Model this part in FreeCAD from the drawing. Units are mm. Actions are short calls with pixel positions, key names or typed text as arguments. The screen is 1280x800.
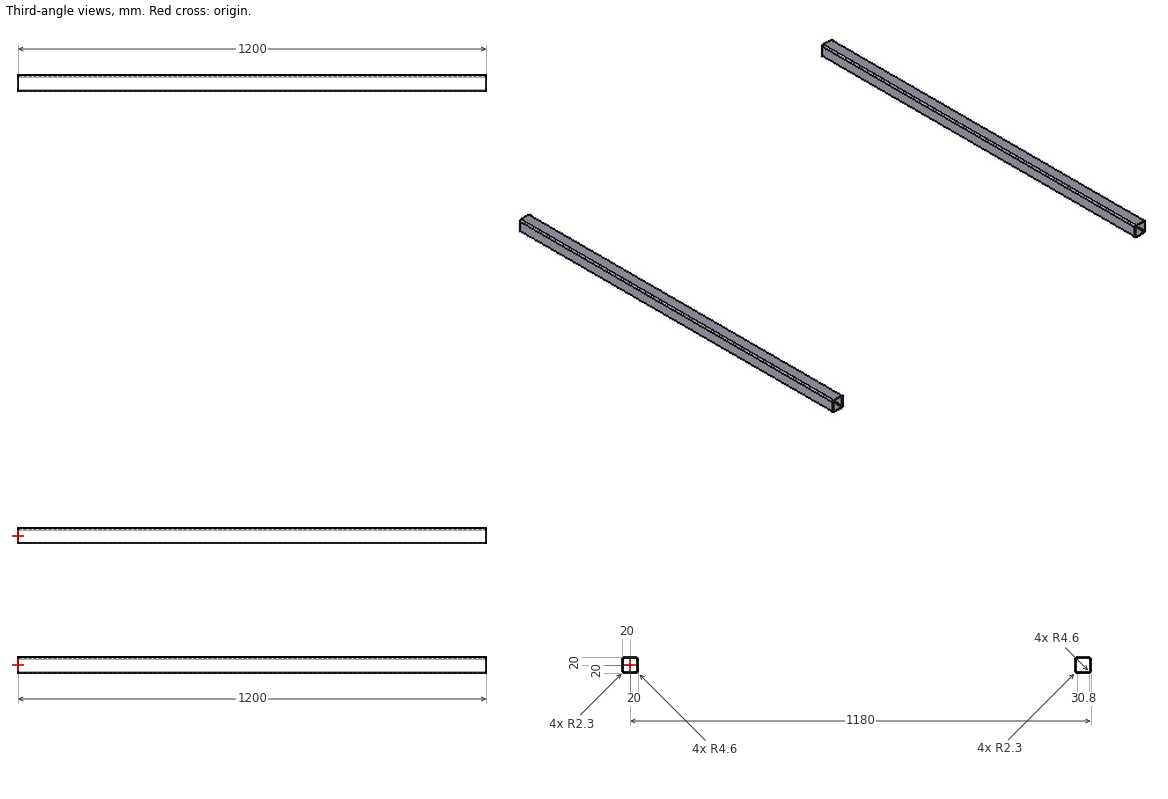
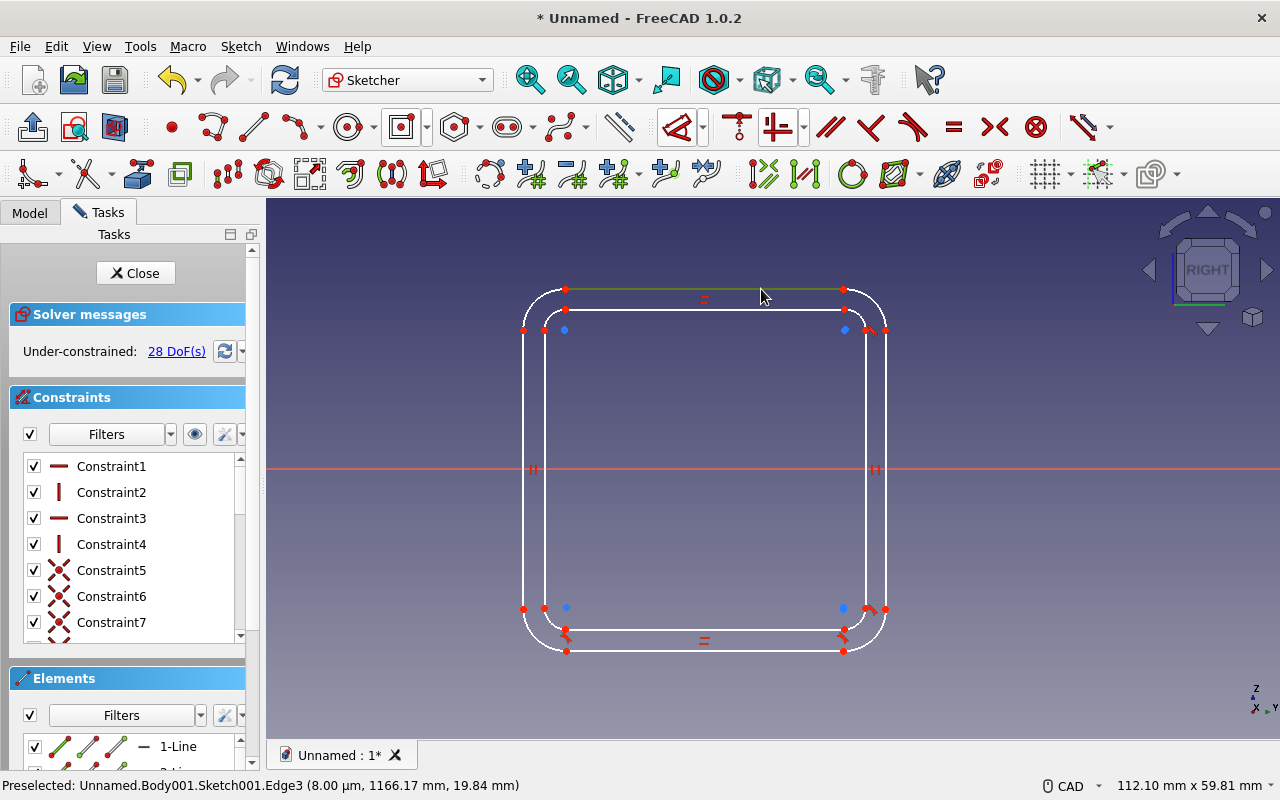
click(881, 311)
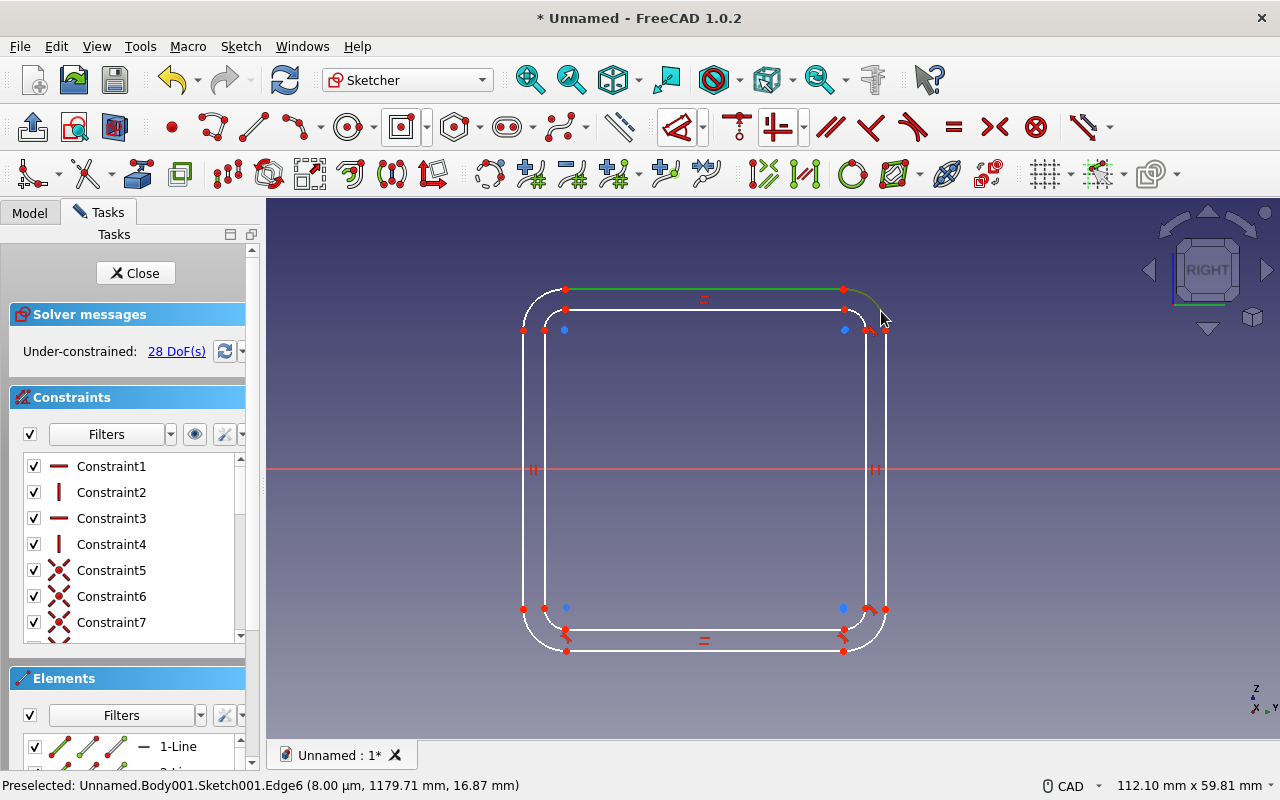
key(t)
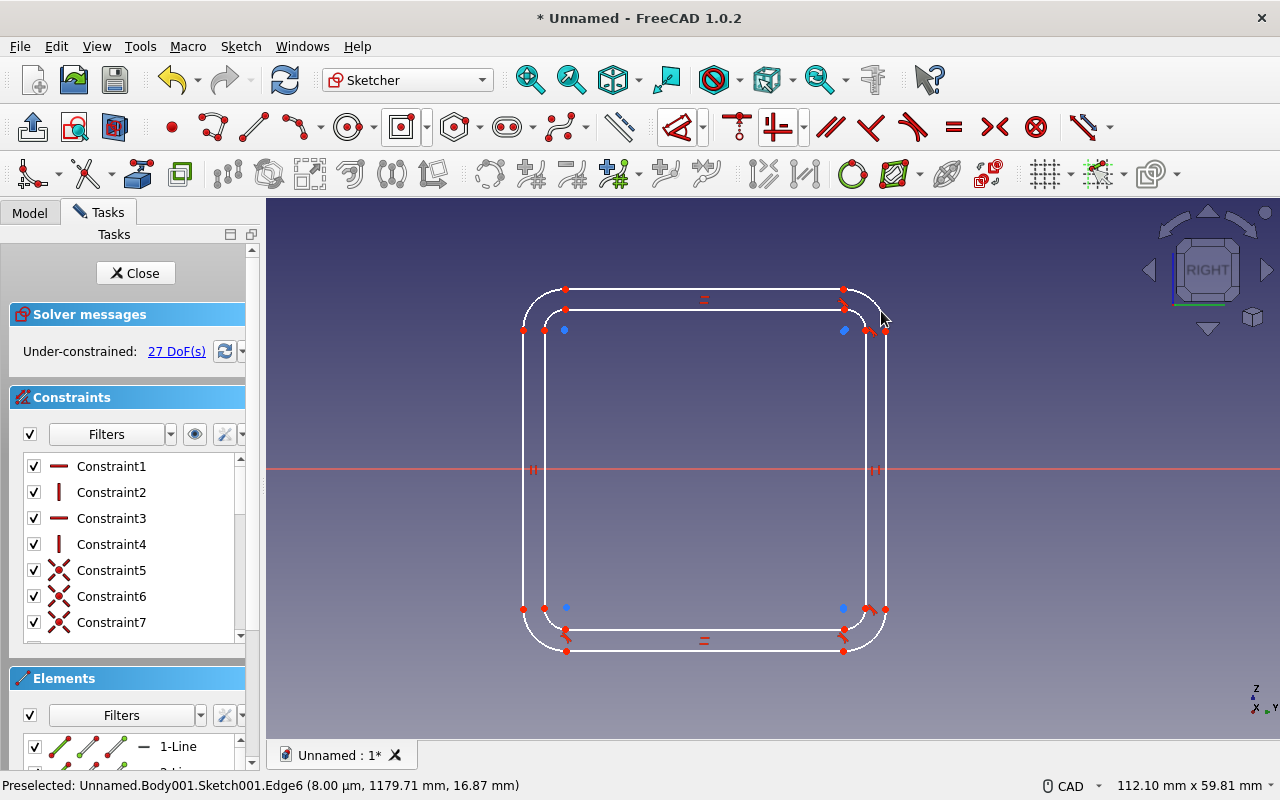
click(761, 289)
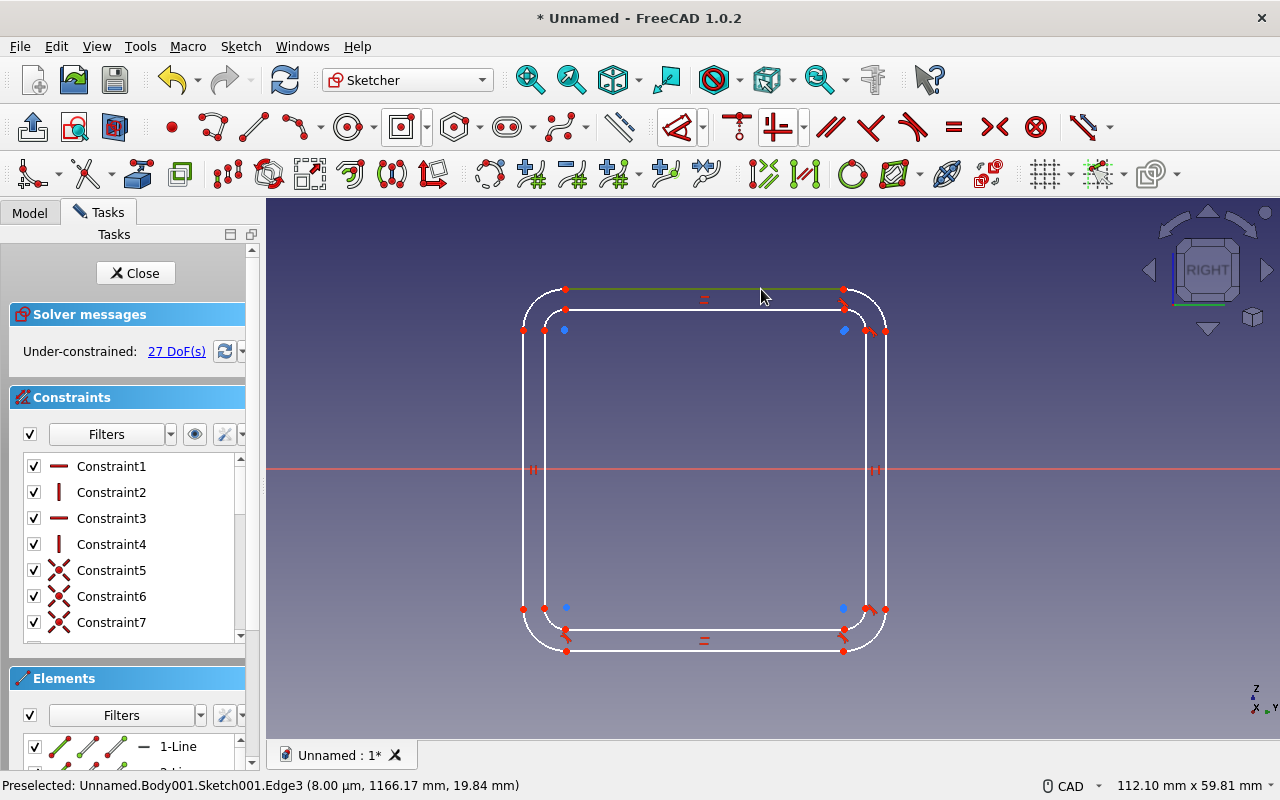
click(547, 293)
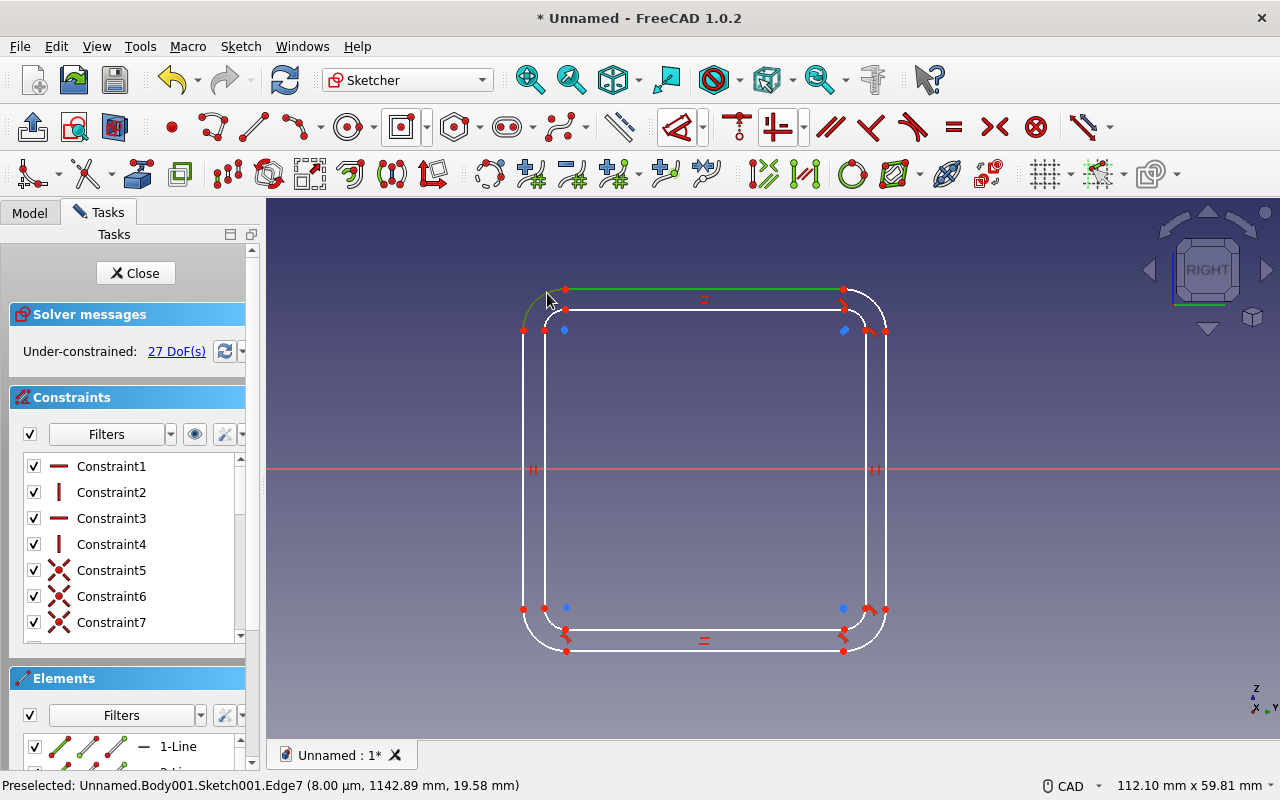
key(t)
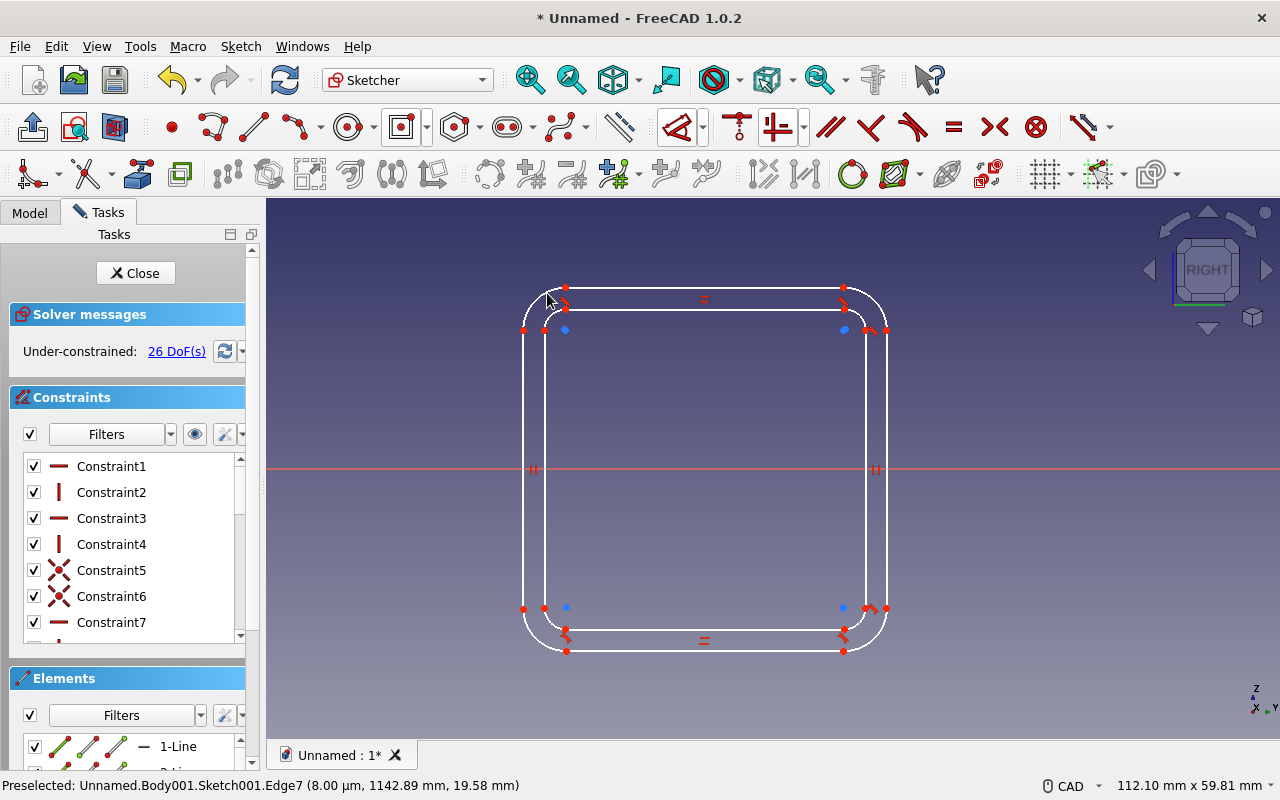
click(523, 414)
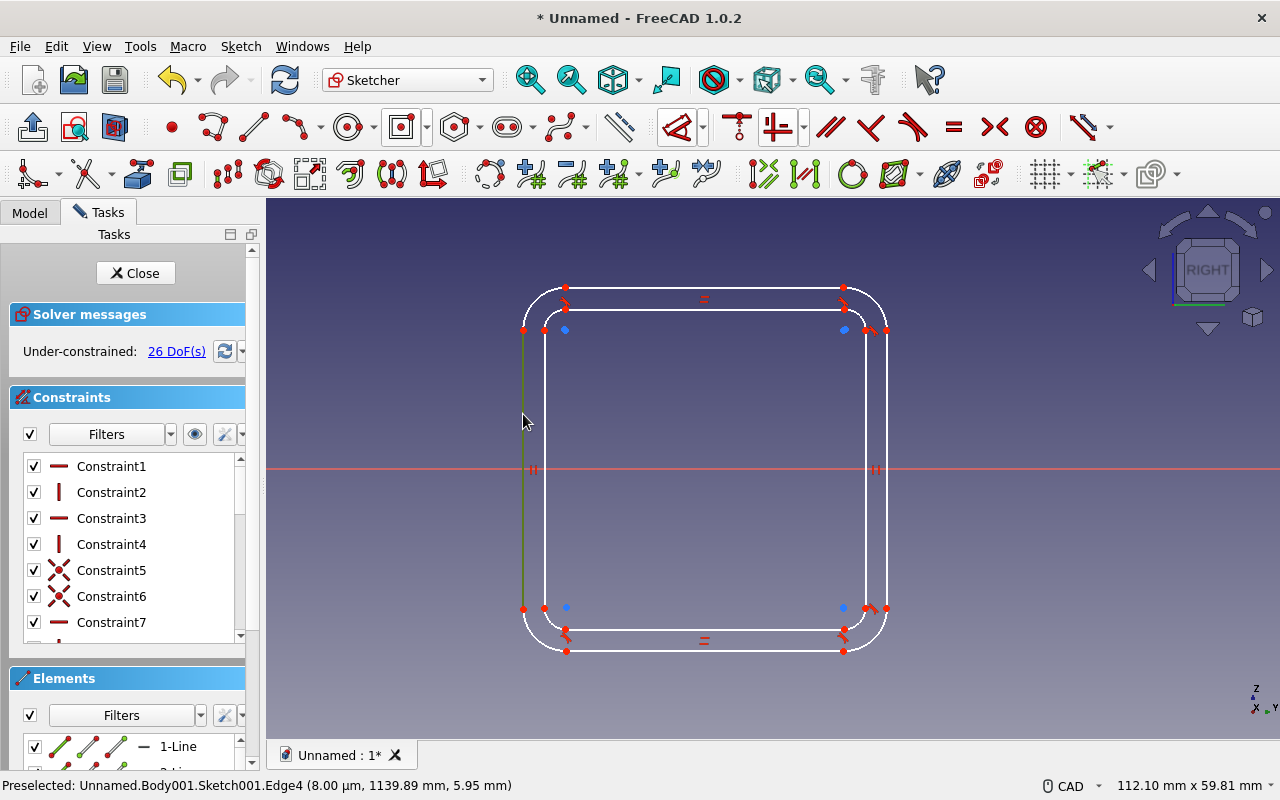
click(547, 292)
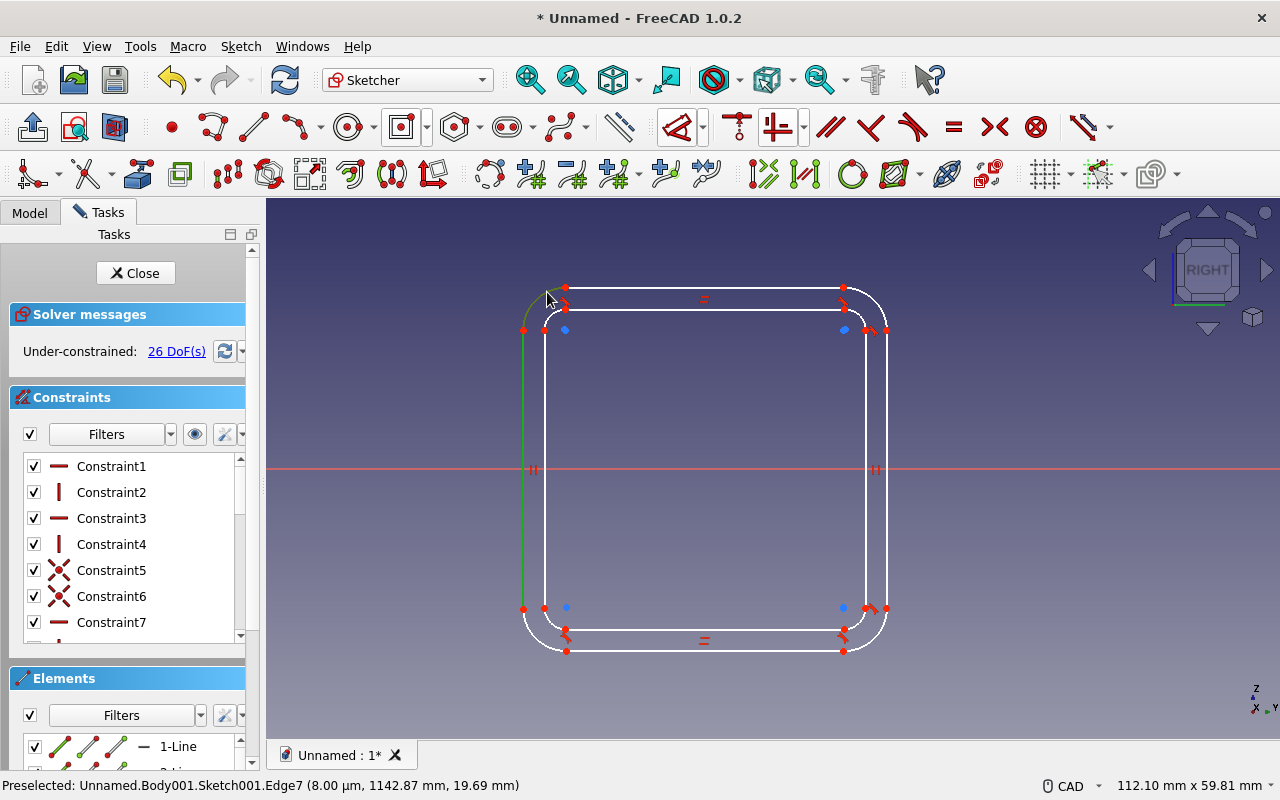
key(t)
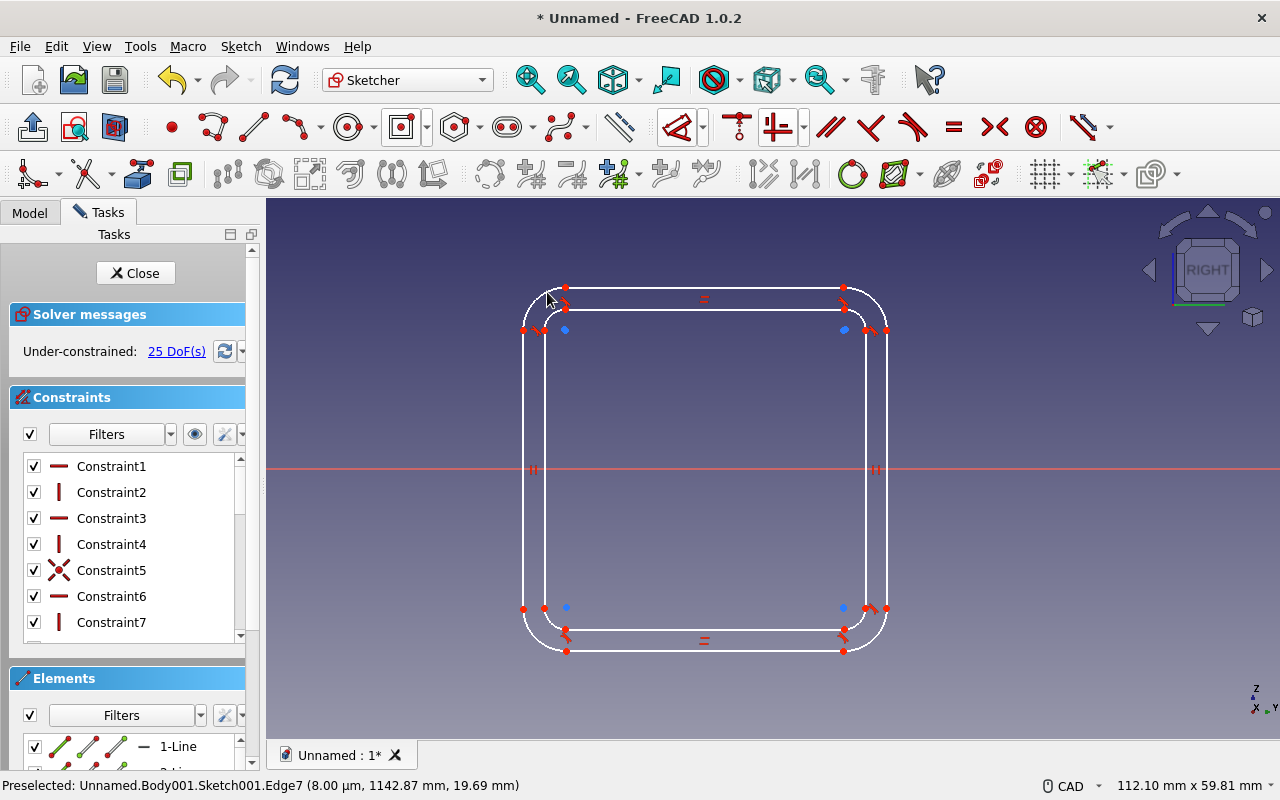
click(523, 414)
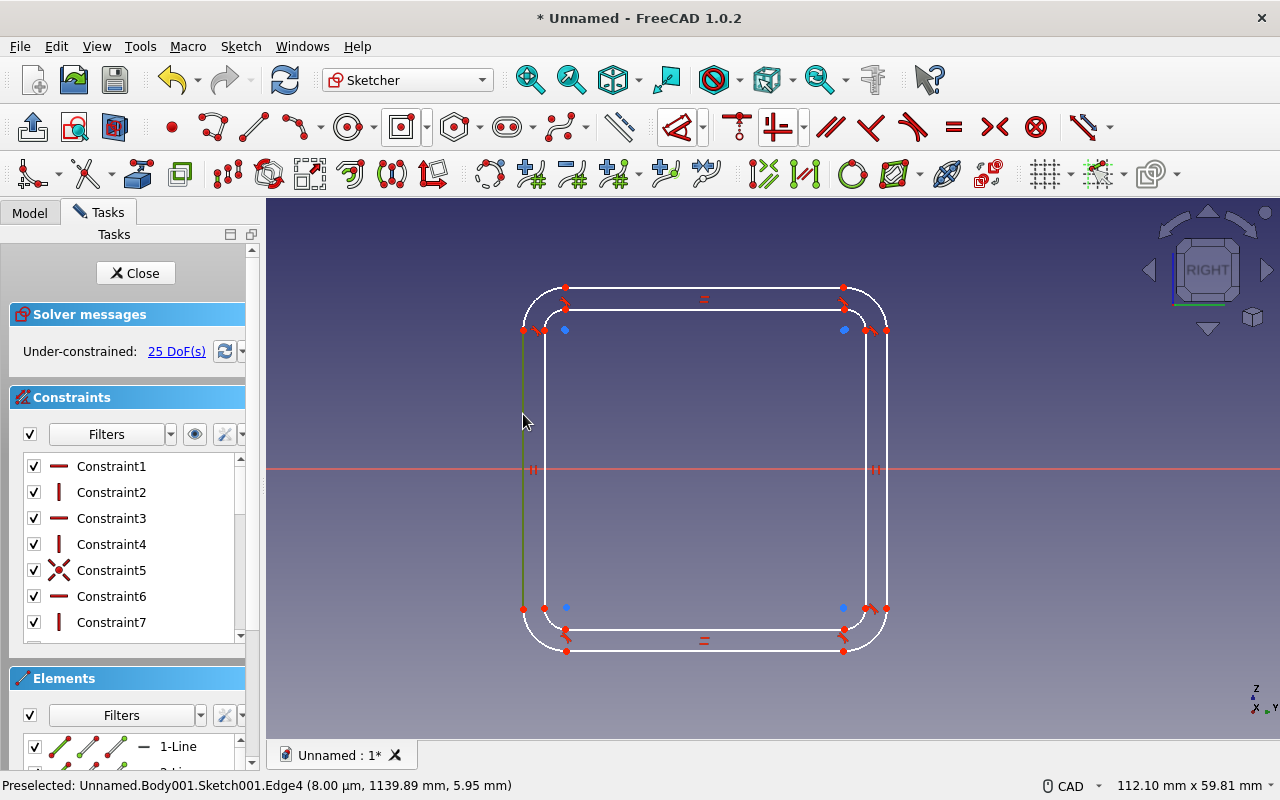
click(528, 628)